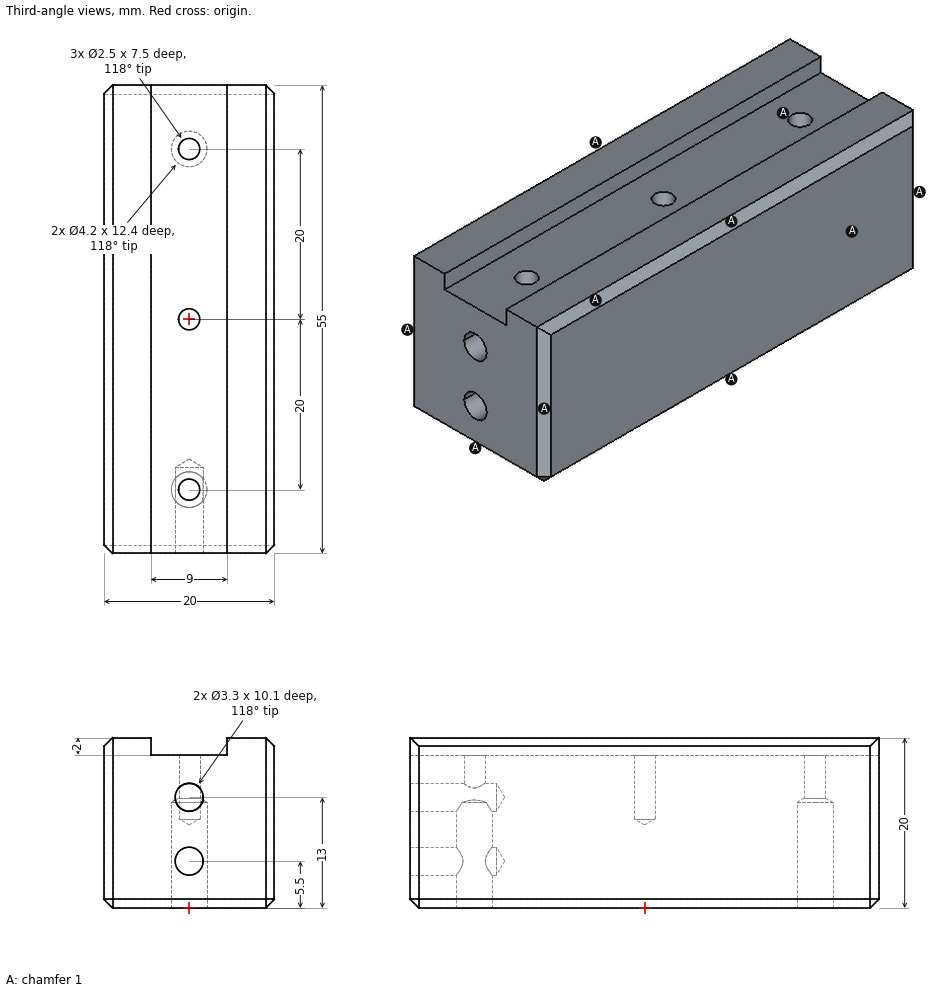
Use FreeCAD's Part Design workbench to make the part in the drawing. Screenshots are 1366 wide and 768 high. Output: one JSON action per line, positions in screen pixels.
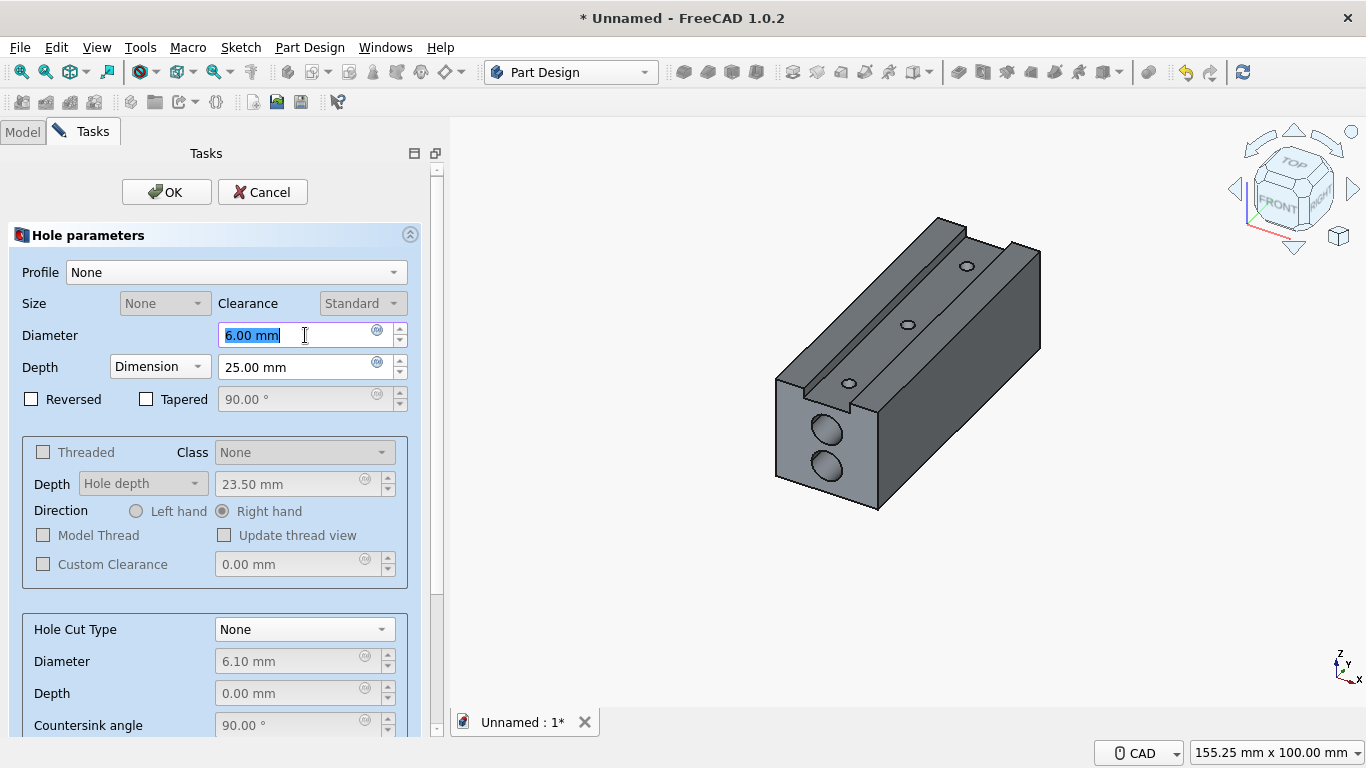
{"action": "type", "text": "3.3"}
{"action": "key", "text": "Tab"}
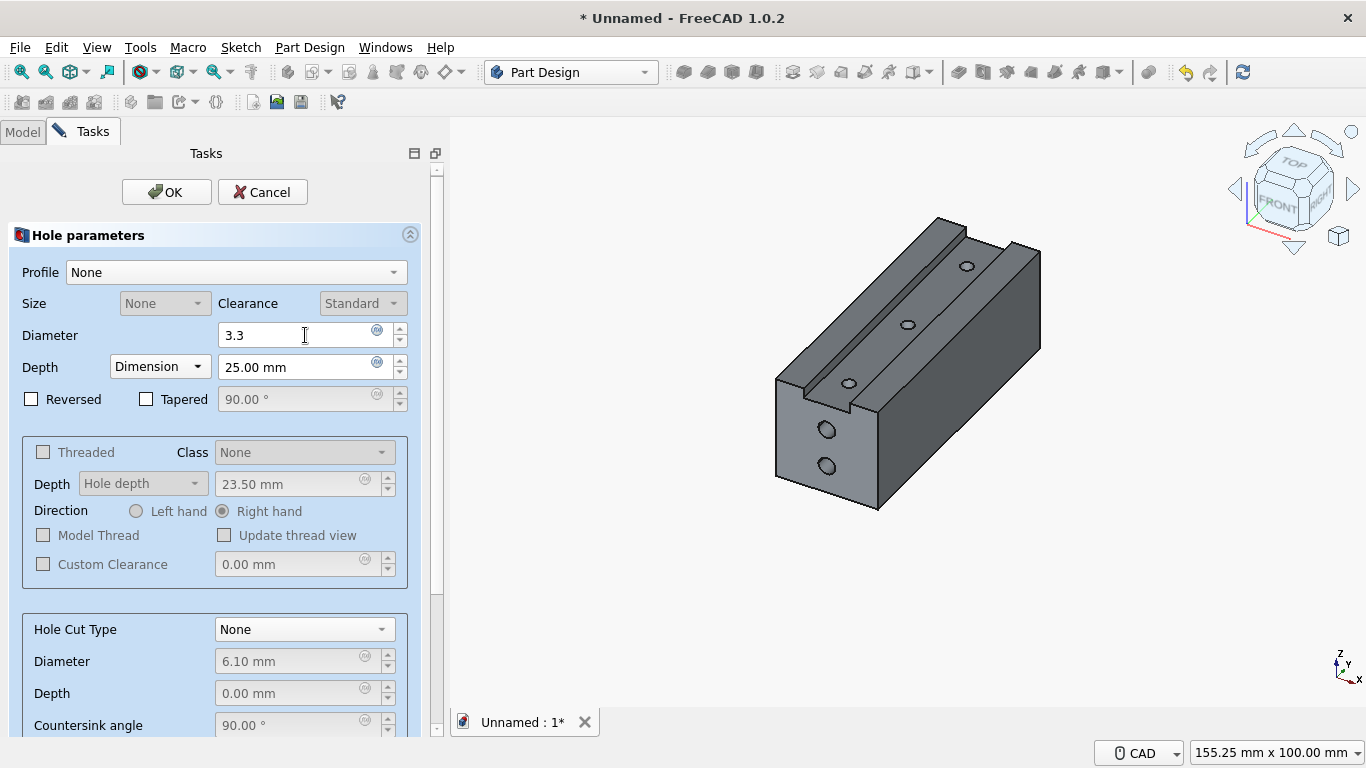
{"action": "triple_click", "coordinate": [305, 367]}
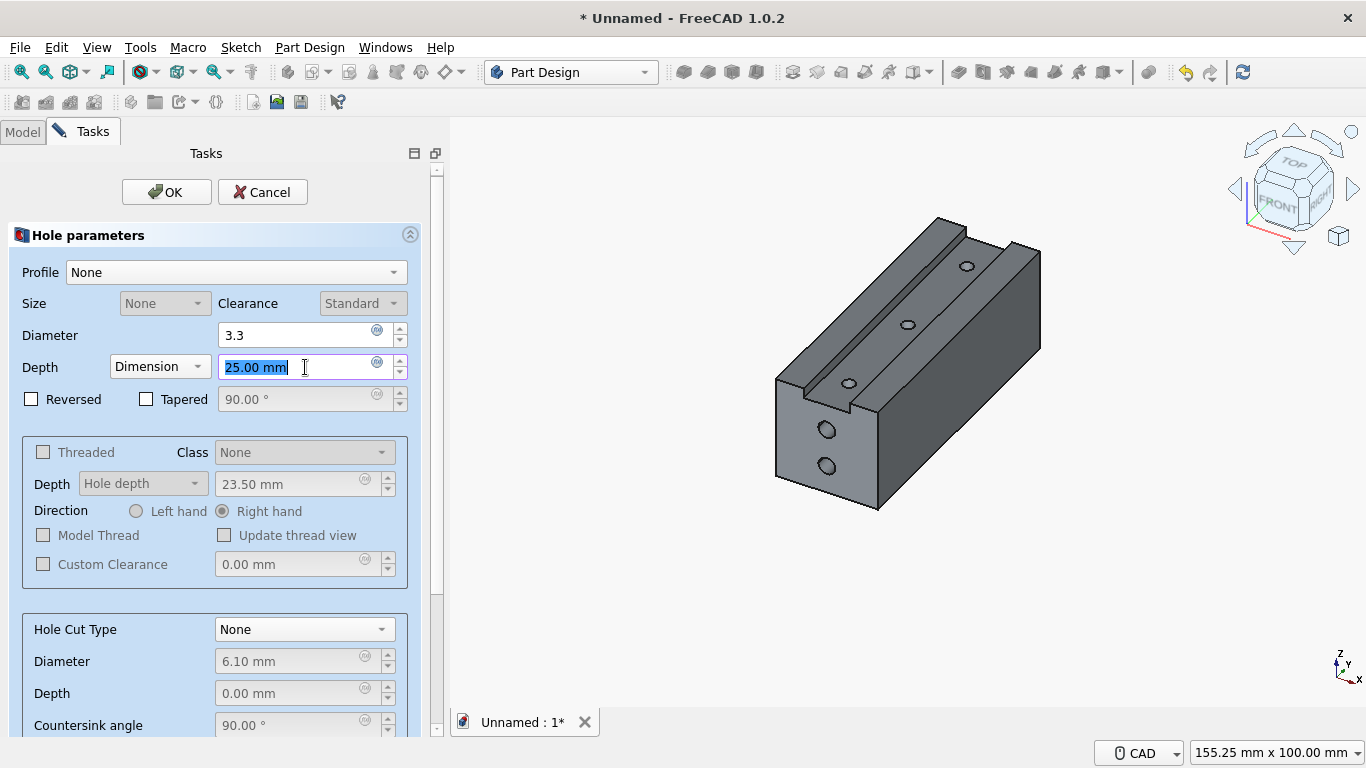
{"action": "type", "text": "10.1"}
{"action": "key", "text": "Tab"}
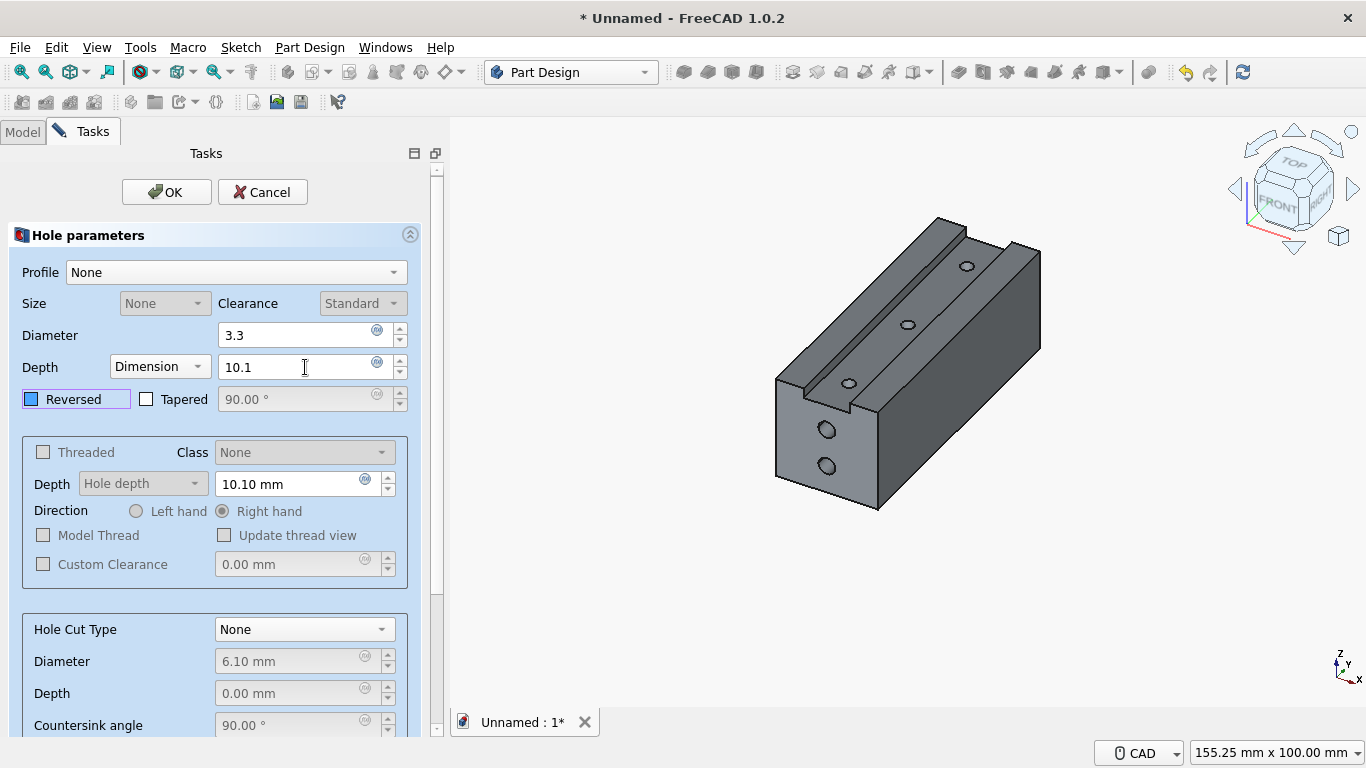
{"action": "left_click", "coordinate": [167, 192]}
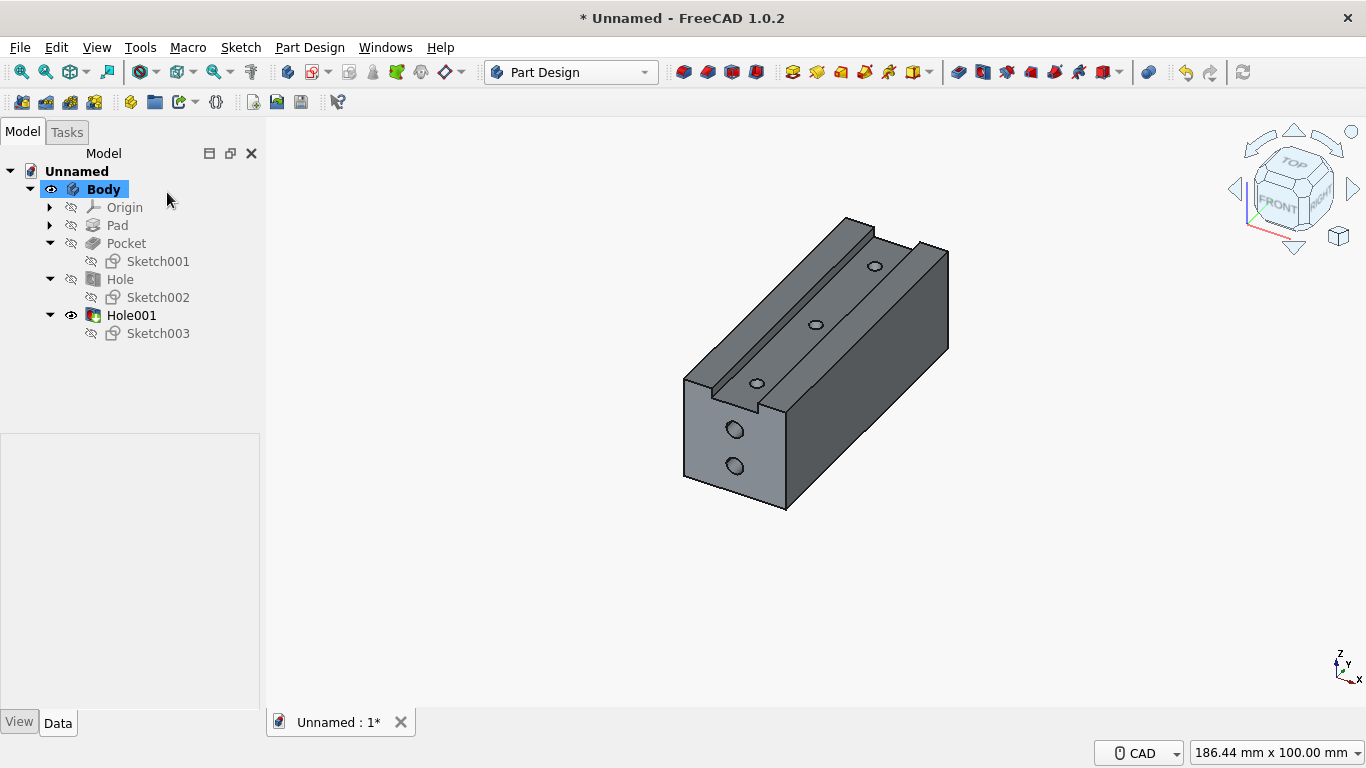
{"action": "key", "text": "5"}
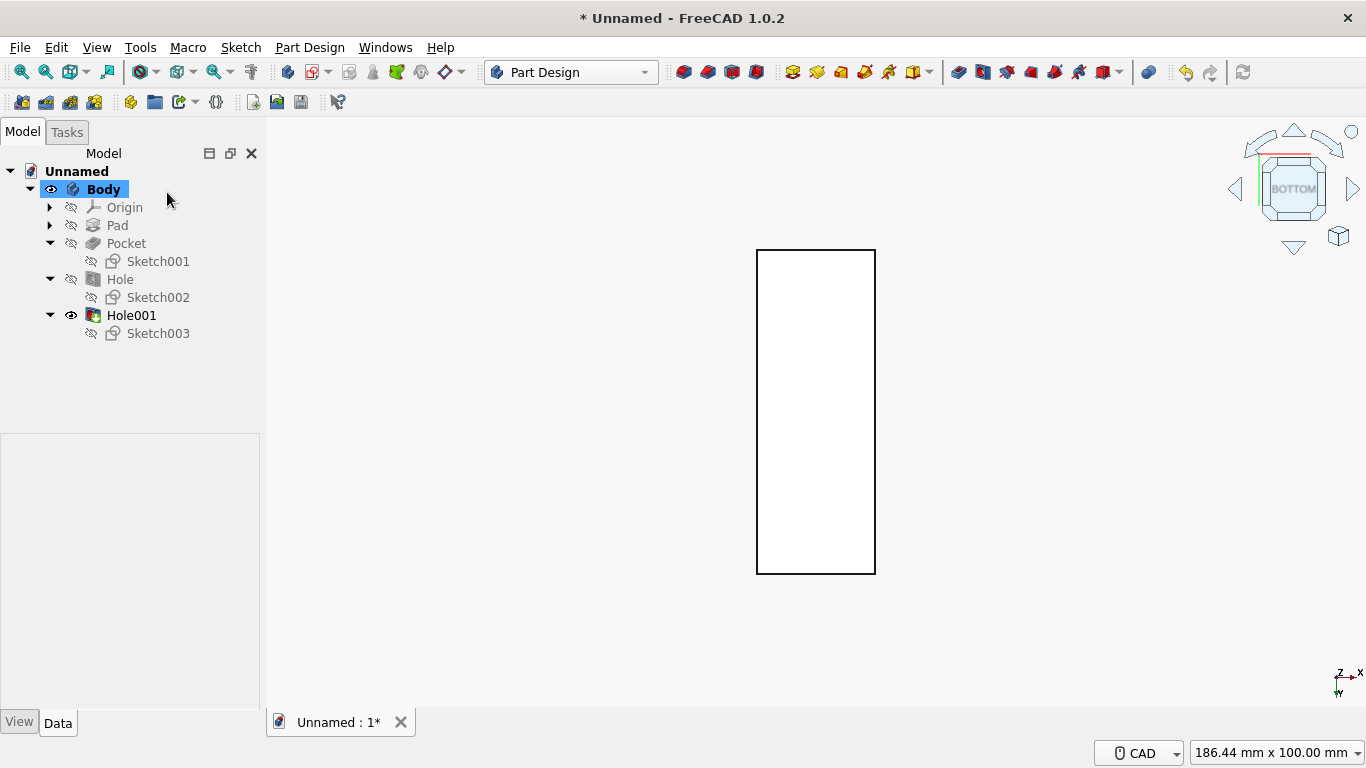
{"action": "left_click", "coordinate": [816, 504]}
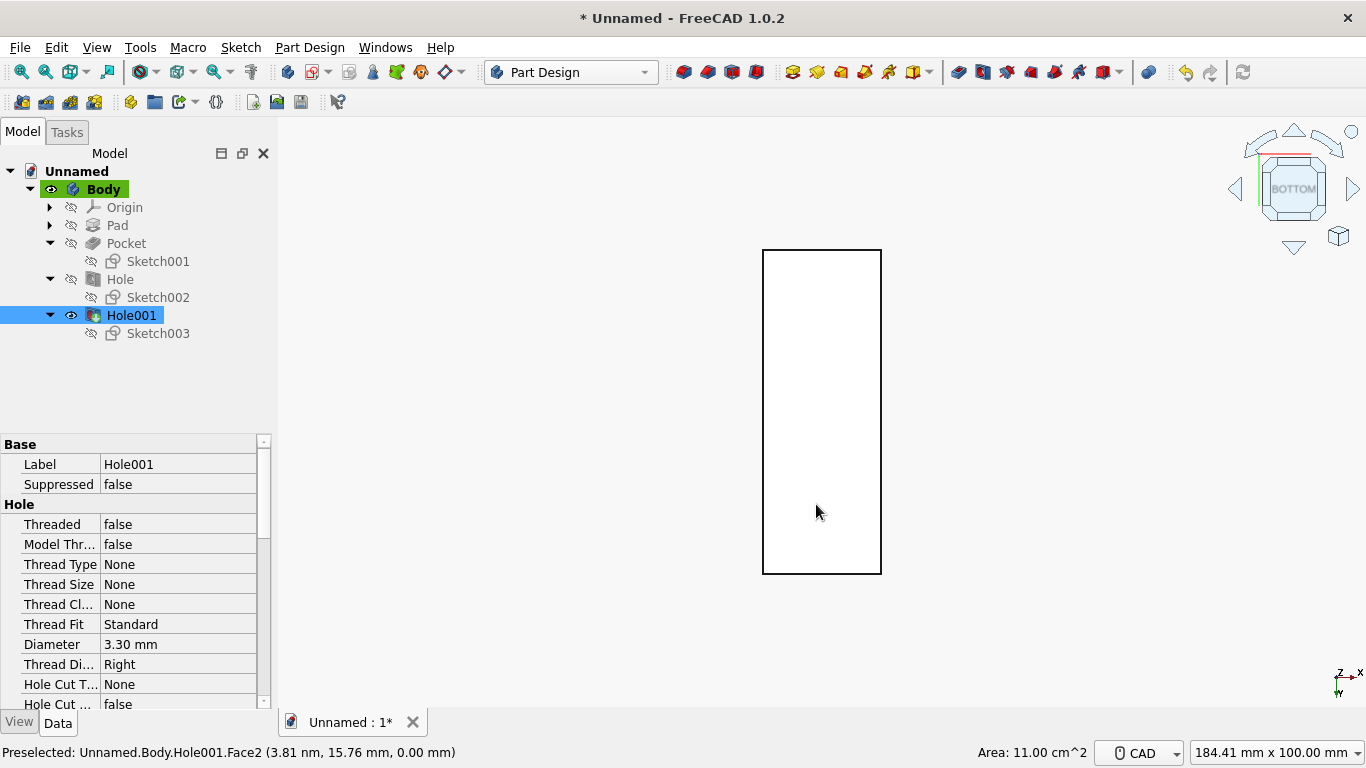
{"action": "left_click", "coordinate": [312, 72]}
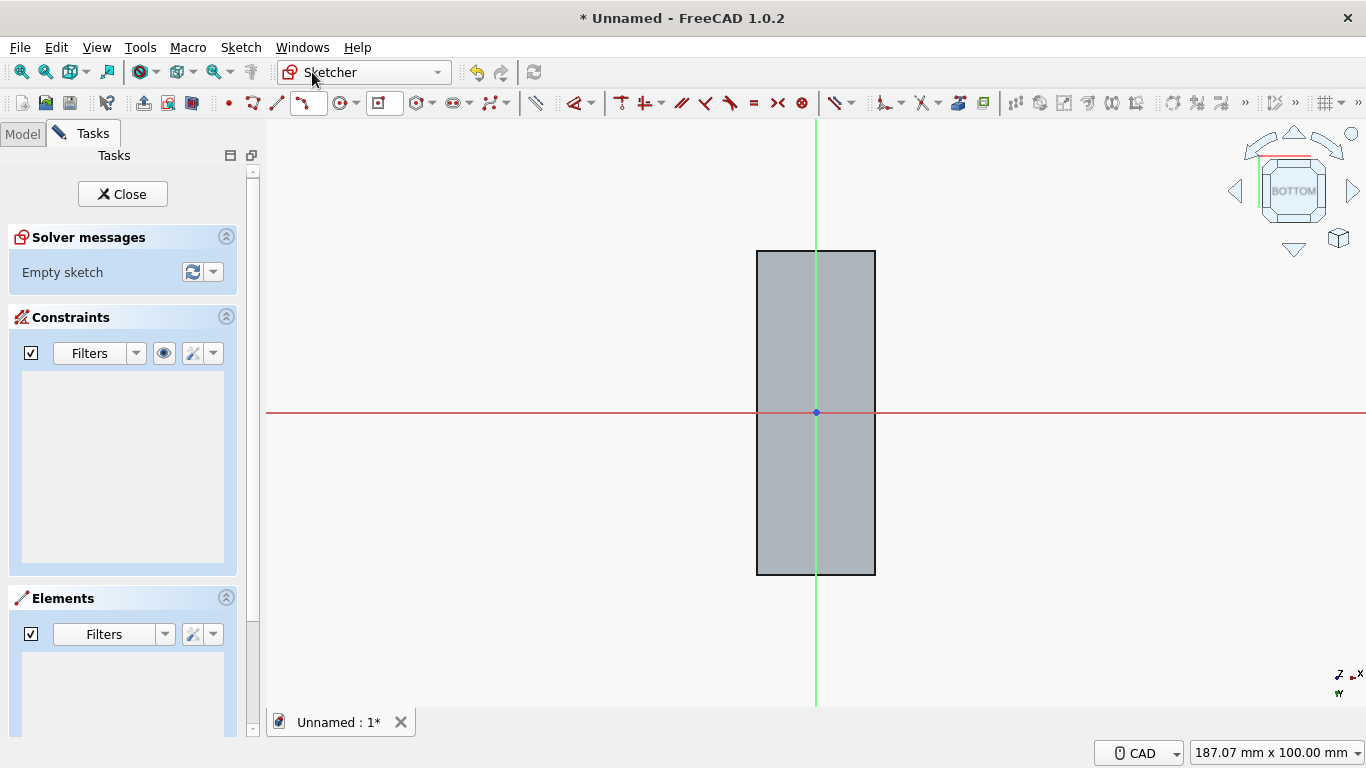
{"action": "scroll", "coordinate": [955, 413], "scroll_direction": "up", "scroll_amount": 2}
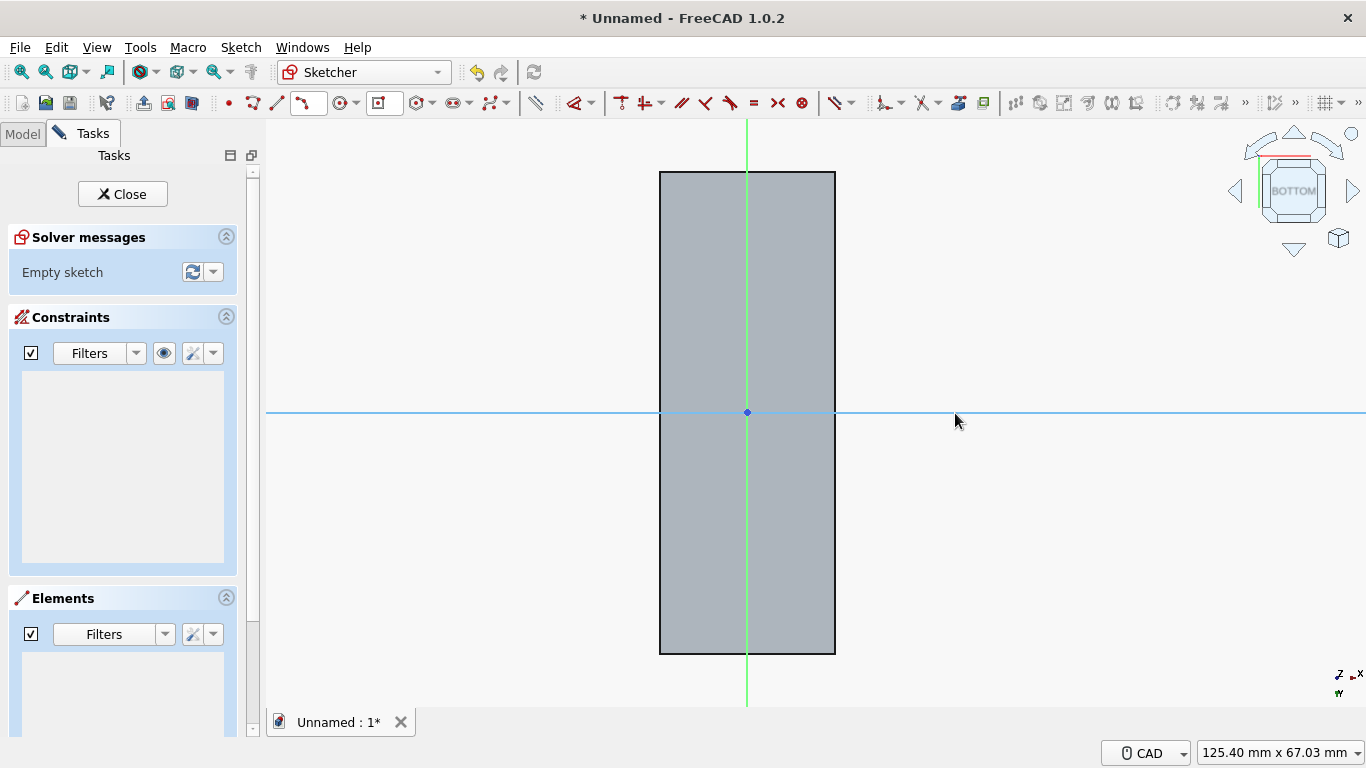
{"action": "key", "text": "g c"}